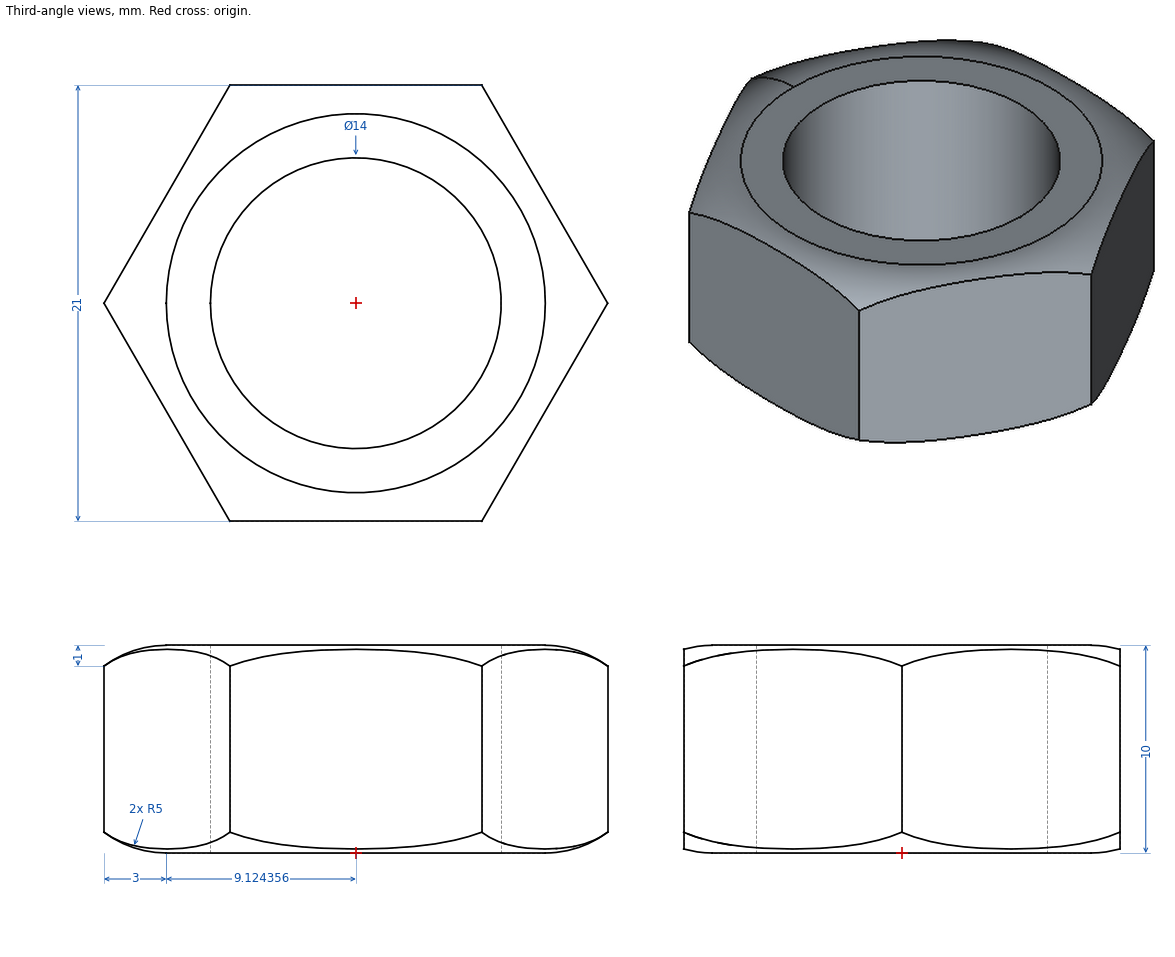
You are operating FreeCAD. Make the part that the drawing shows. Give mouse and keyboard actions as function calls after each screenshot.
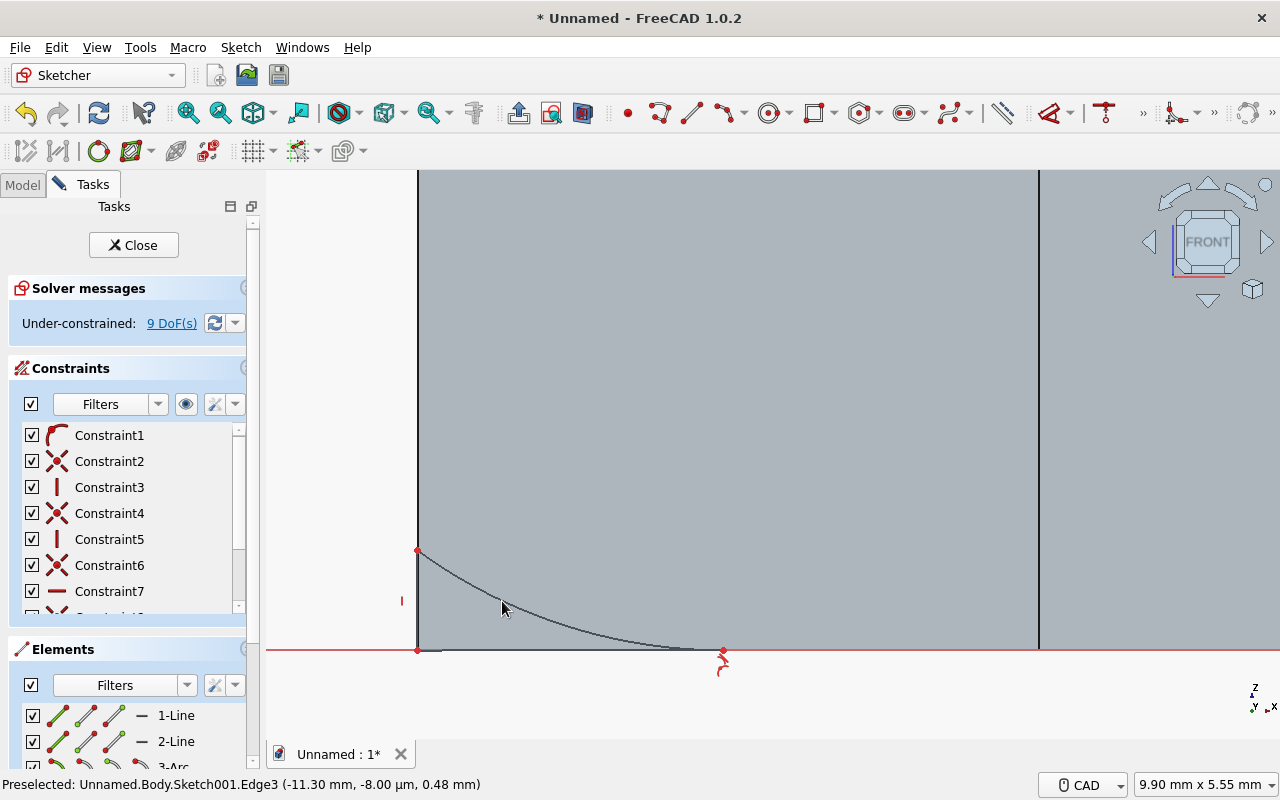
scroll(510, 639, down, 5)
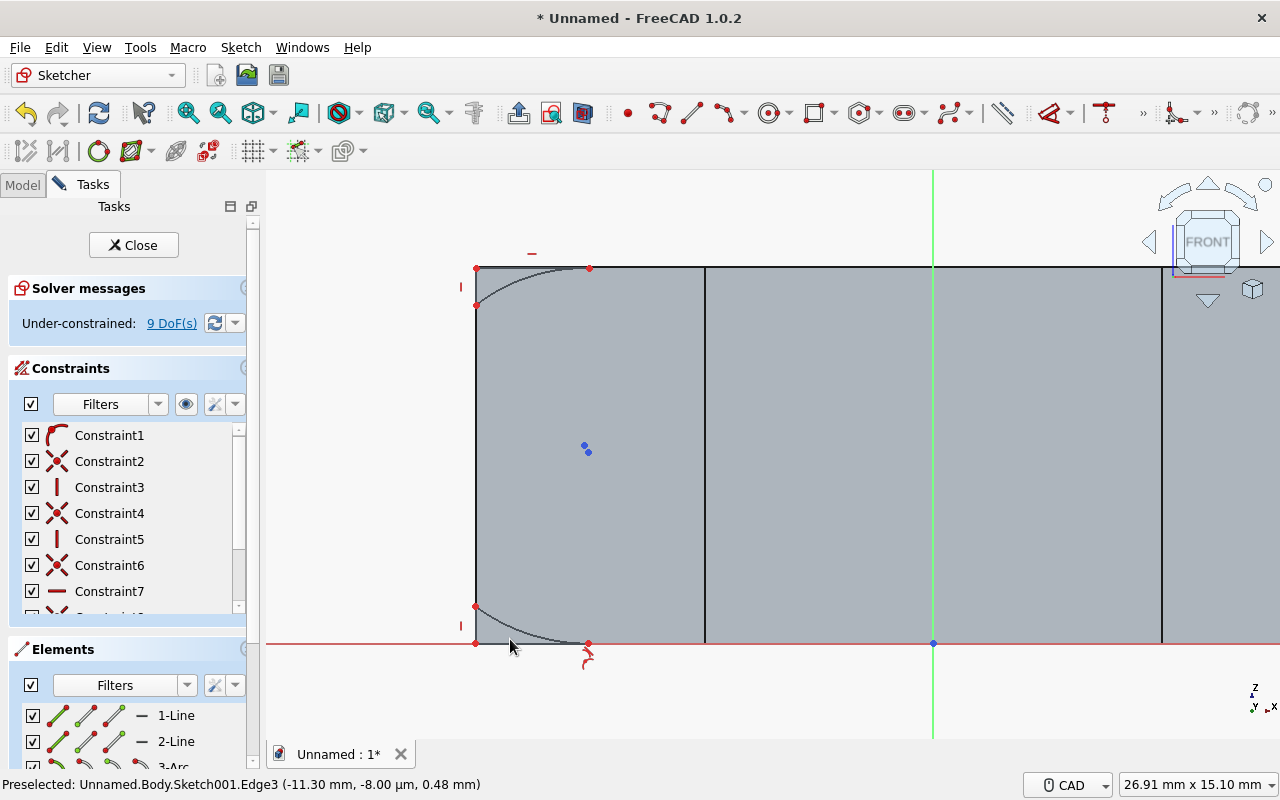
click(510, 268)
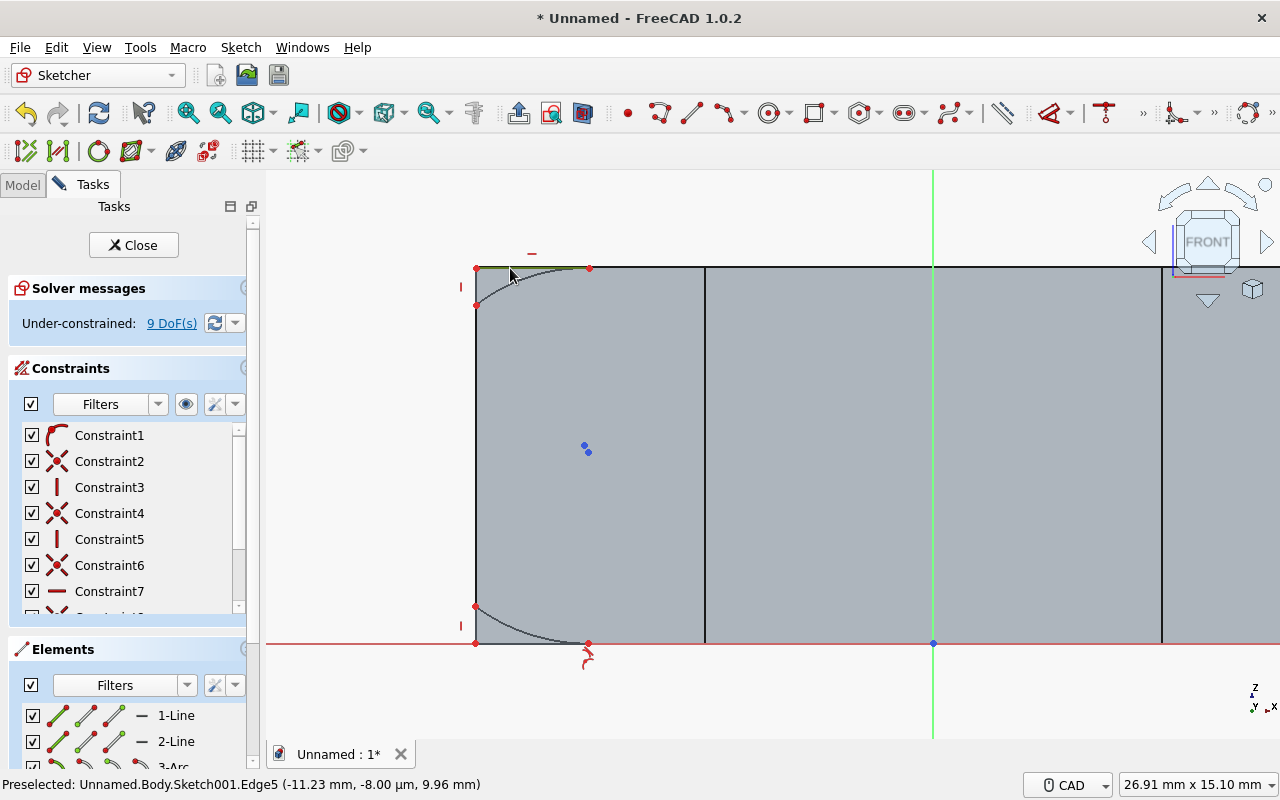
click(507, 286)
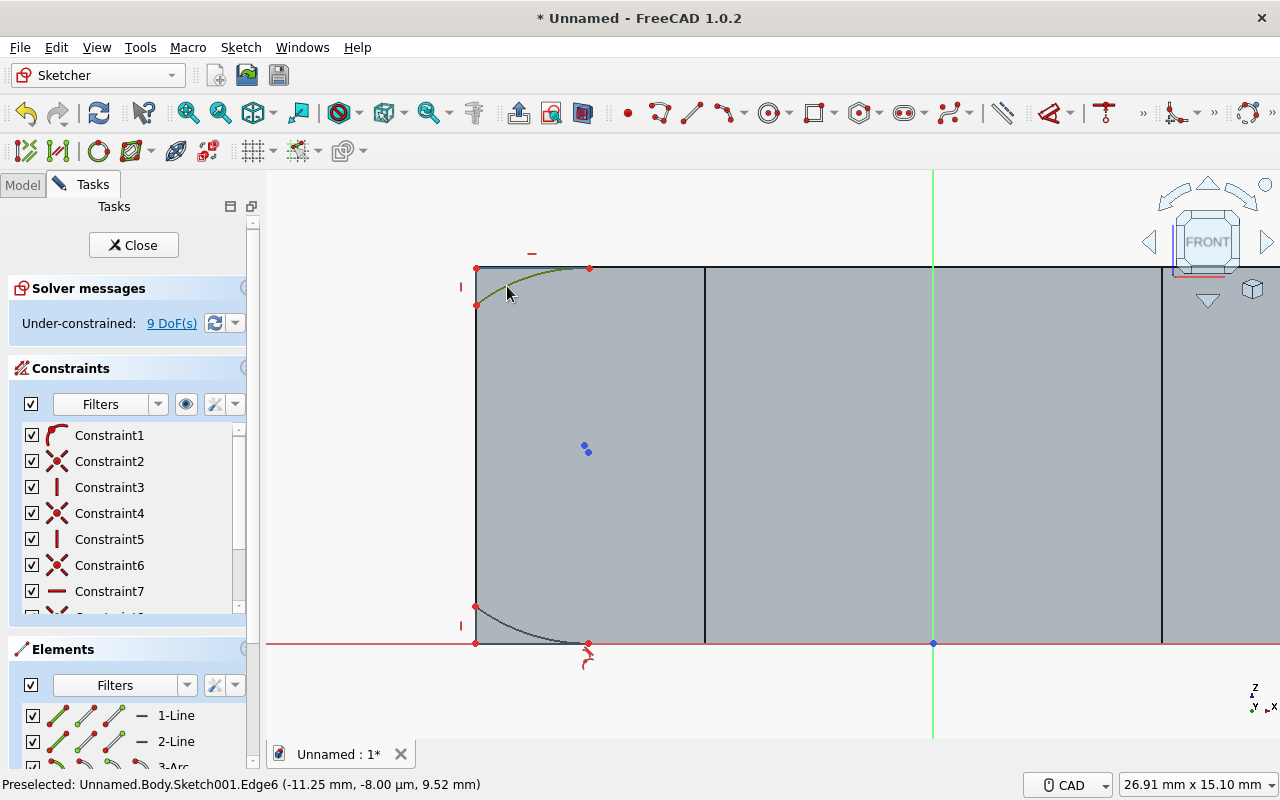
key(t)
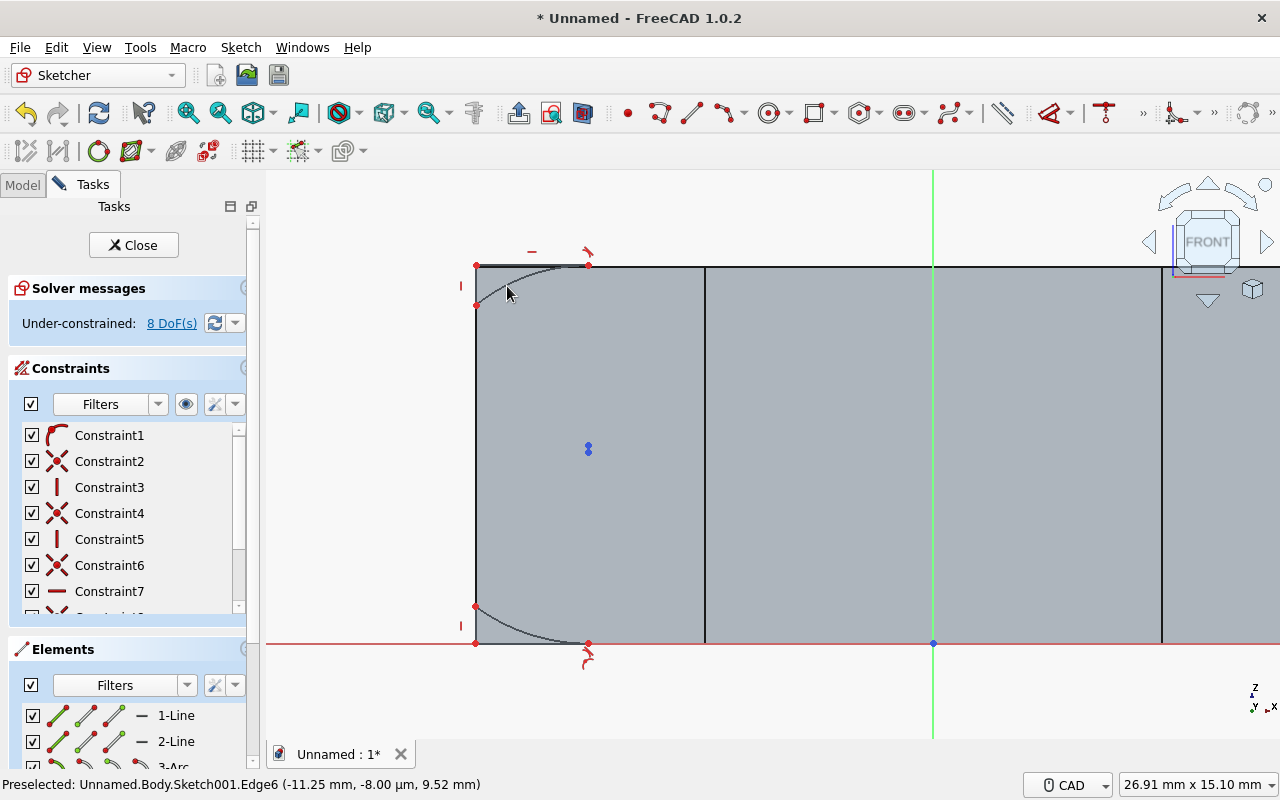
click(510, 644)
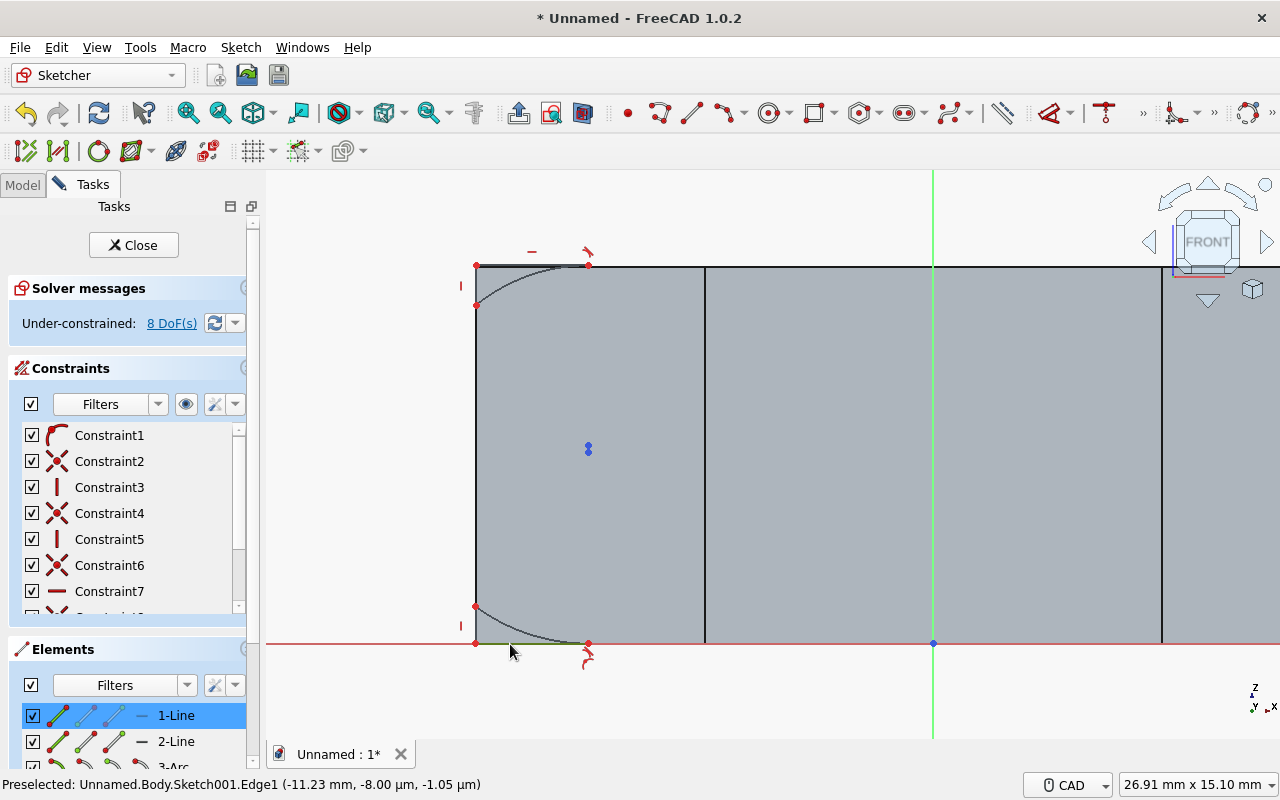
key(h)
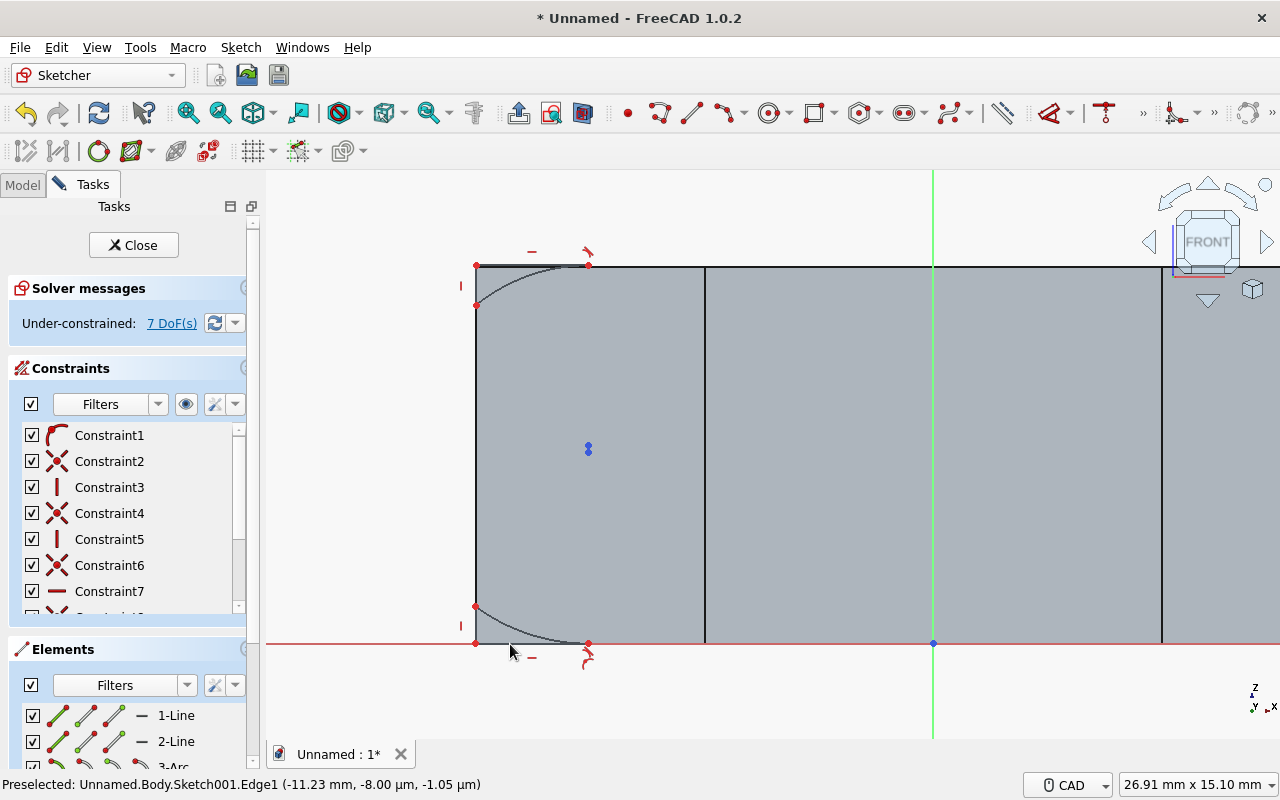
click(507, 625)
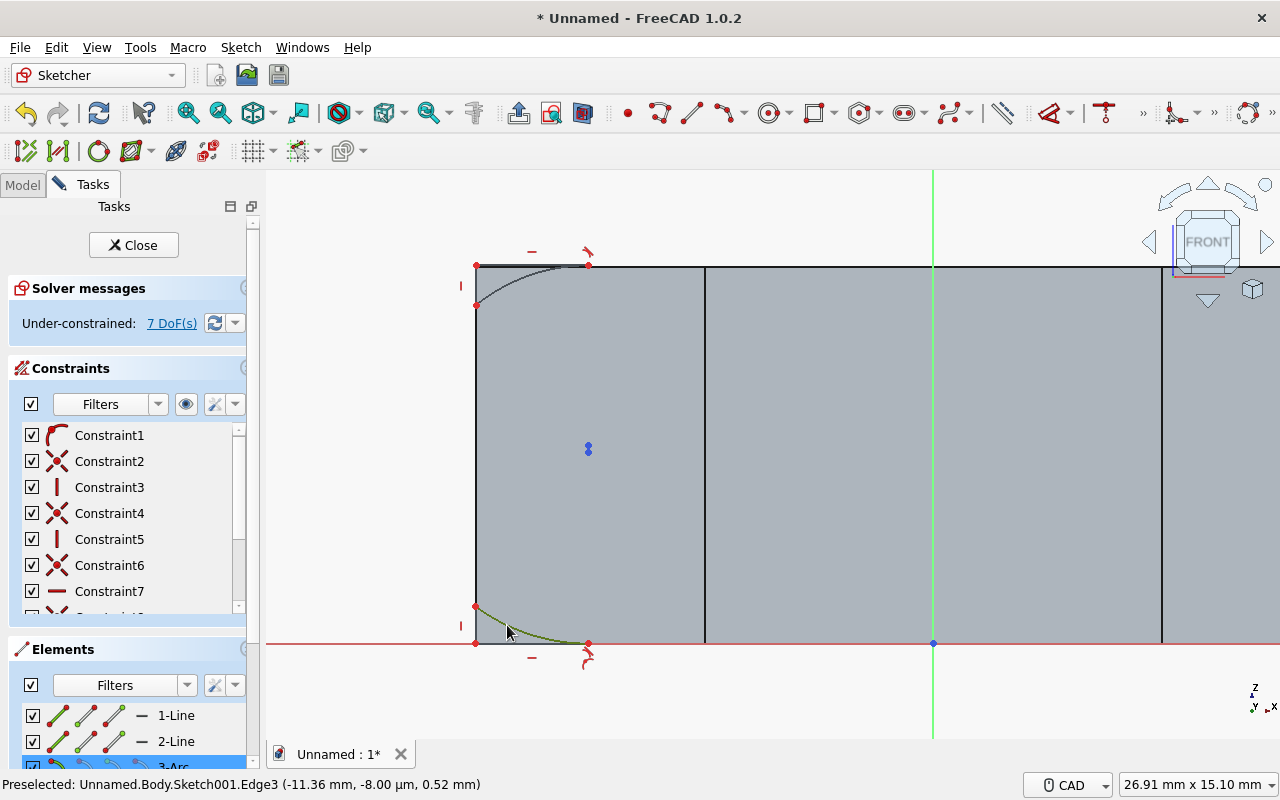
click(507, 285)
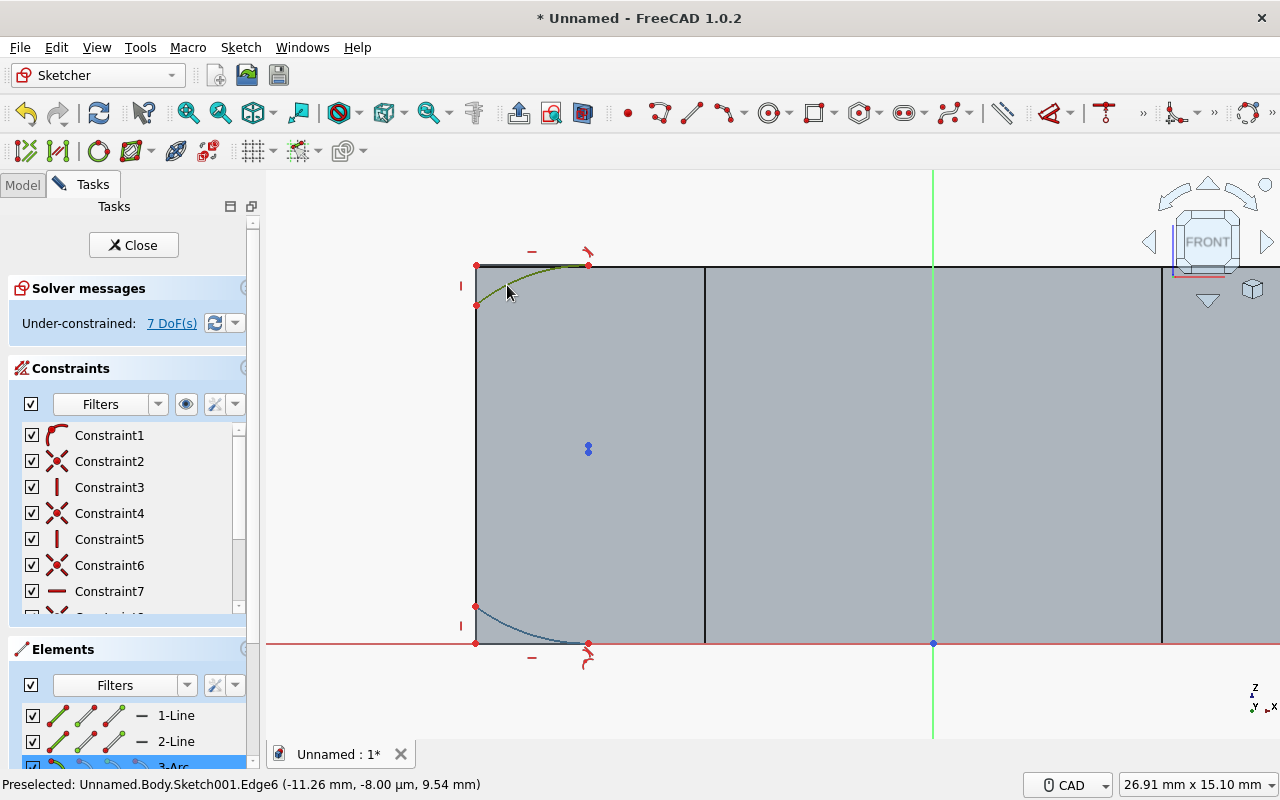
key(c)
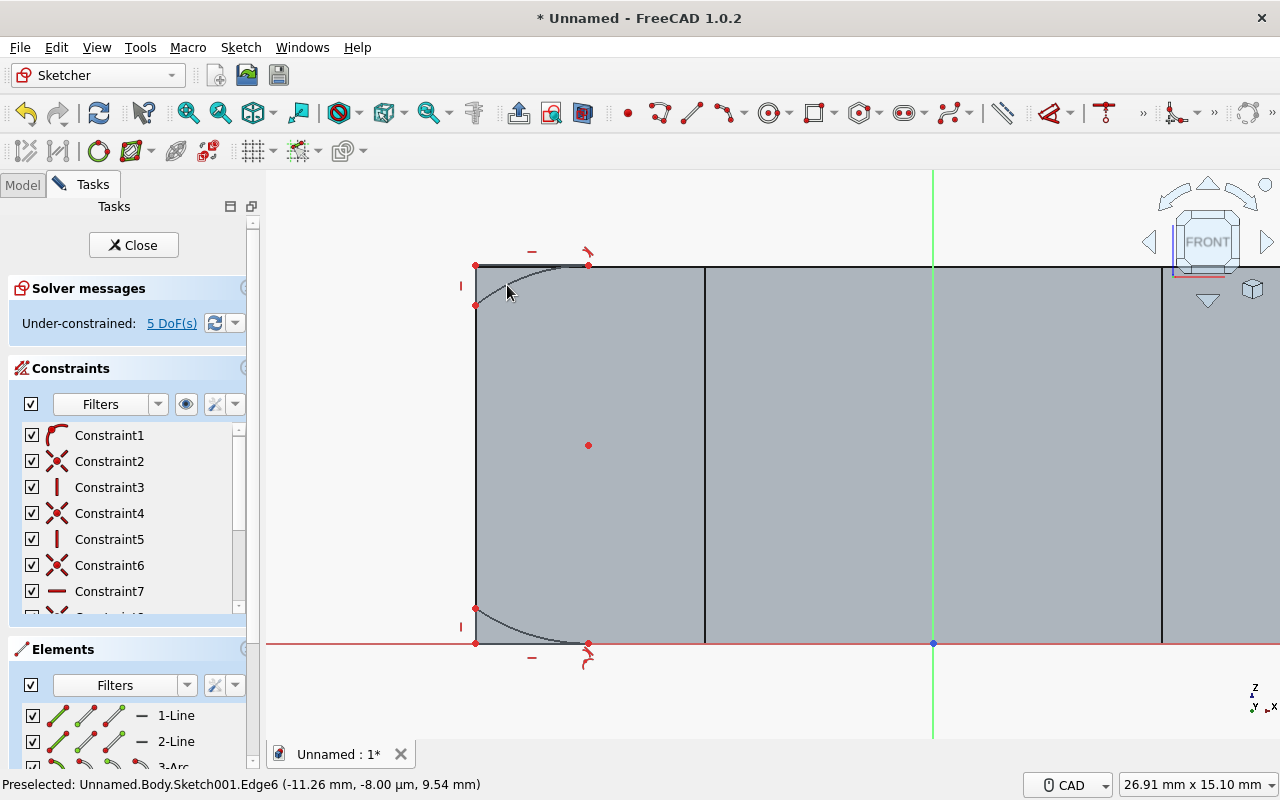
click(507, 626)